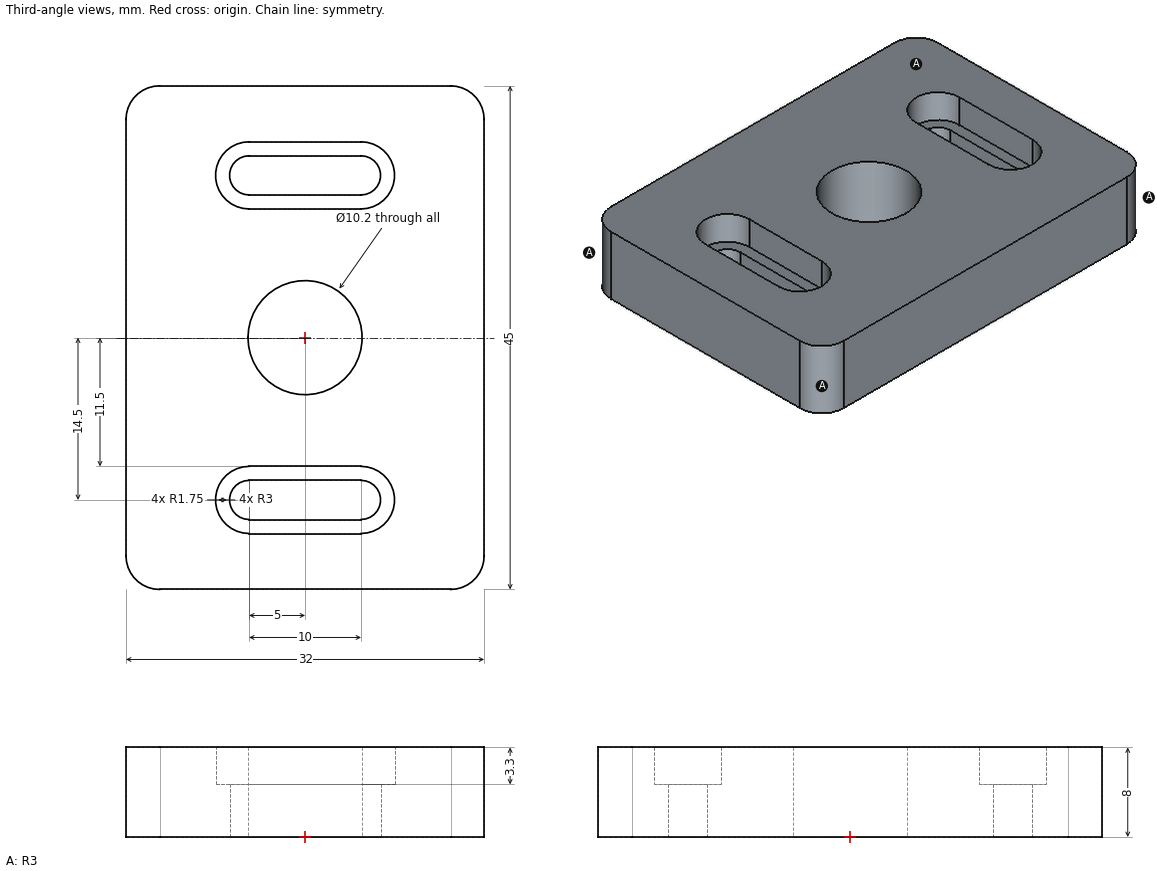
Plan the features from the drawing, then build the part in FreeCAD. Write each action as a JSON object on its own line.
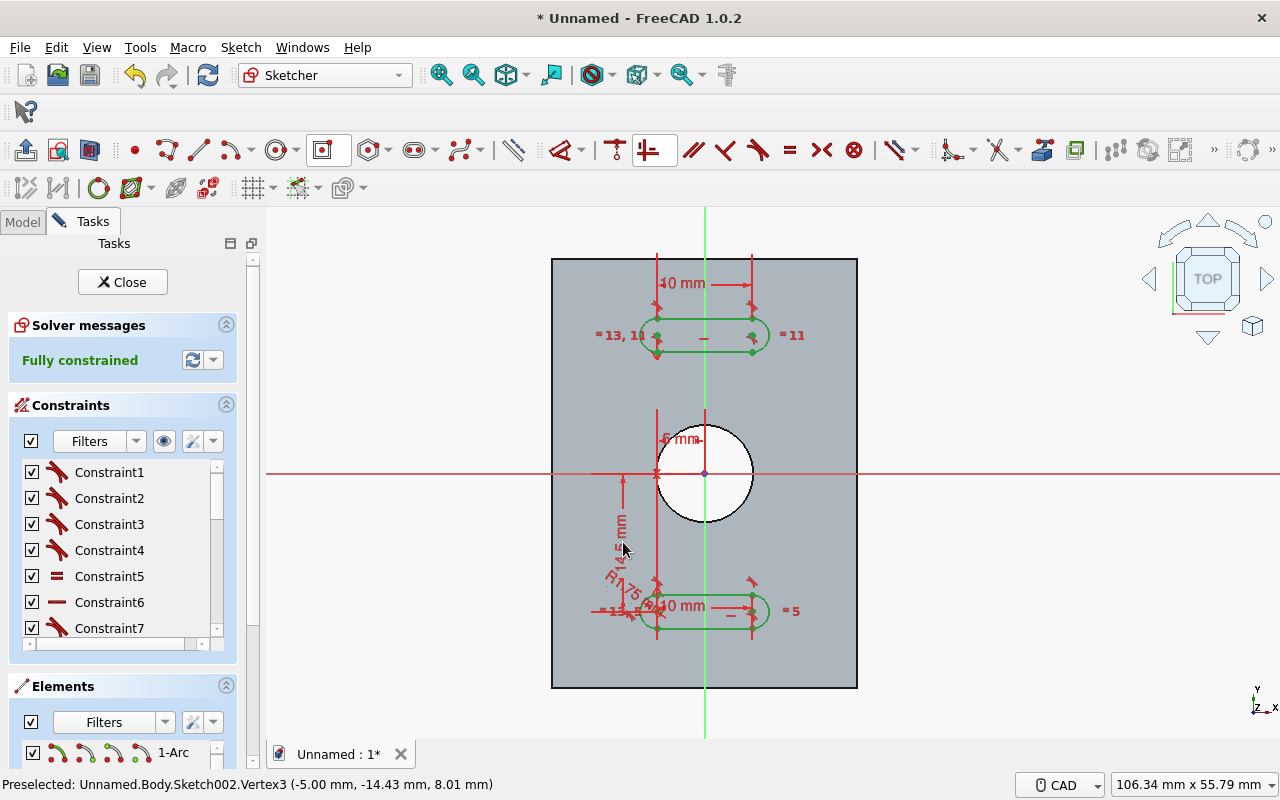
{"action": "left_click", "coordinate": [123, 282]}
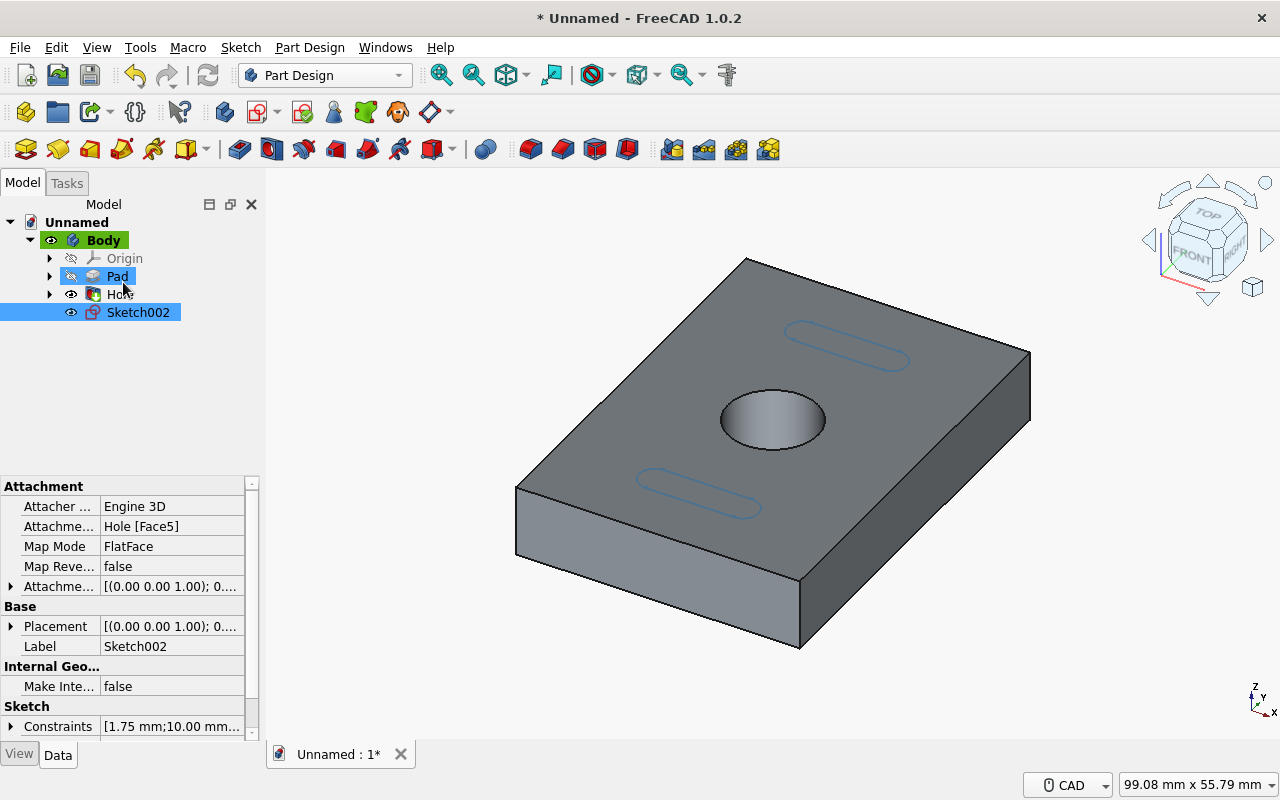
{"action": "left_click", "coordinate": [240, 150]}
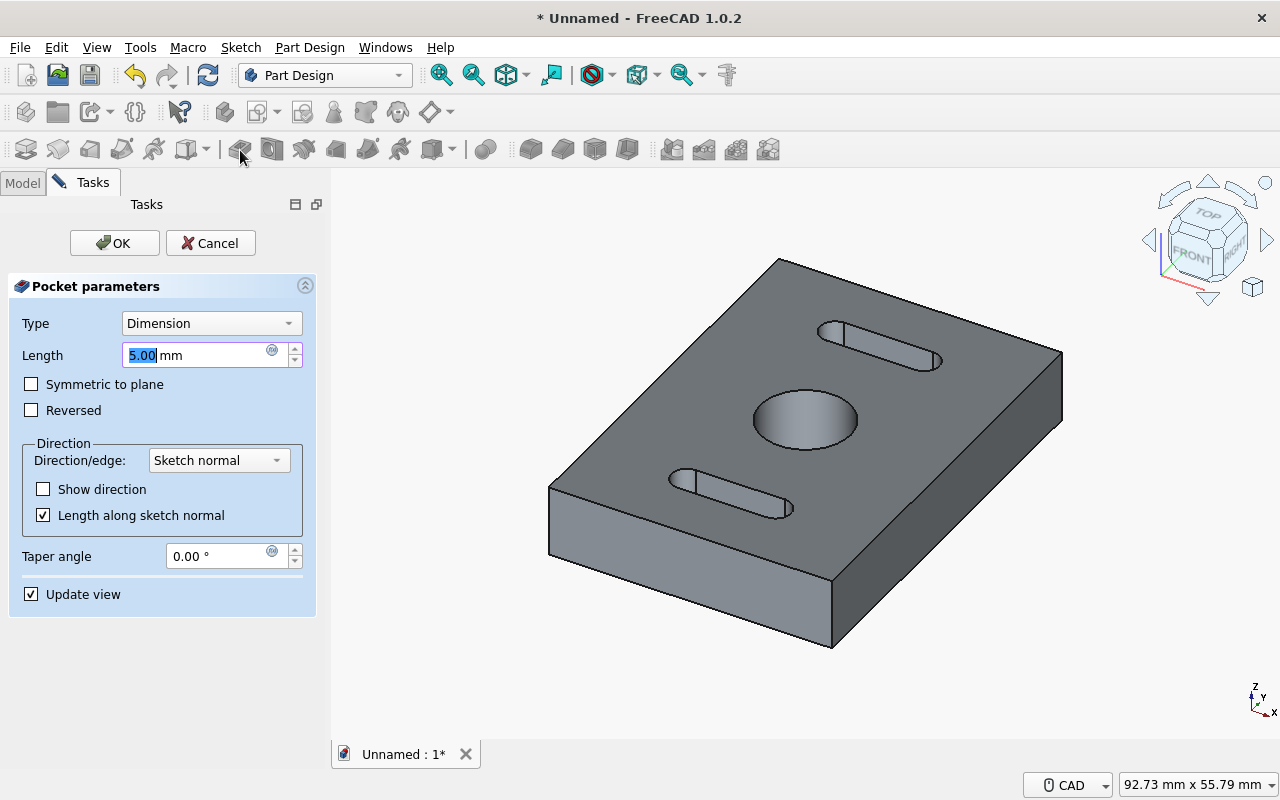
{"action": "left_click", "coordinate": [212, 324]}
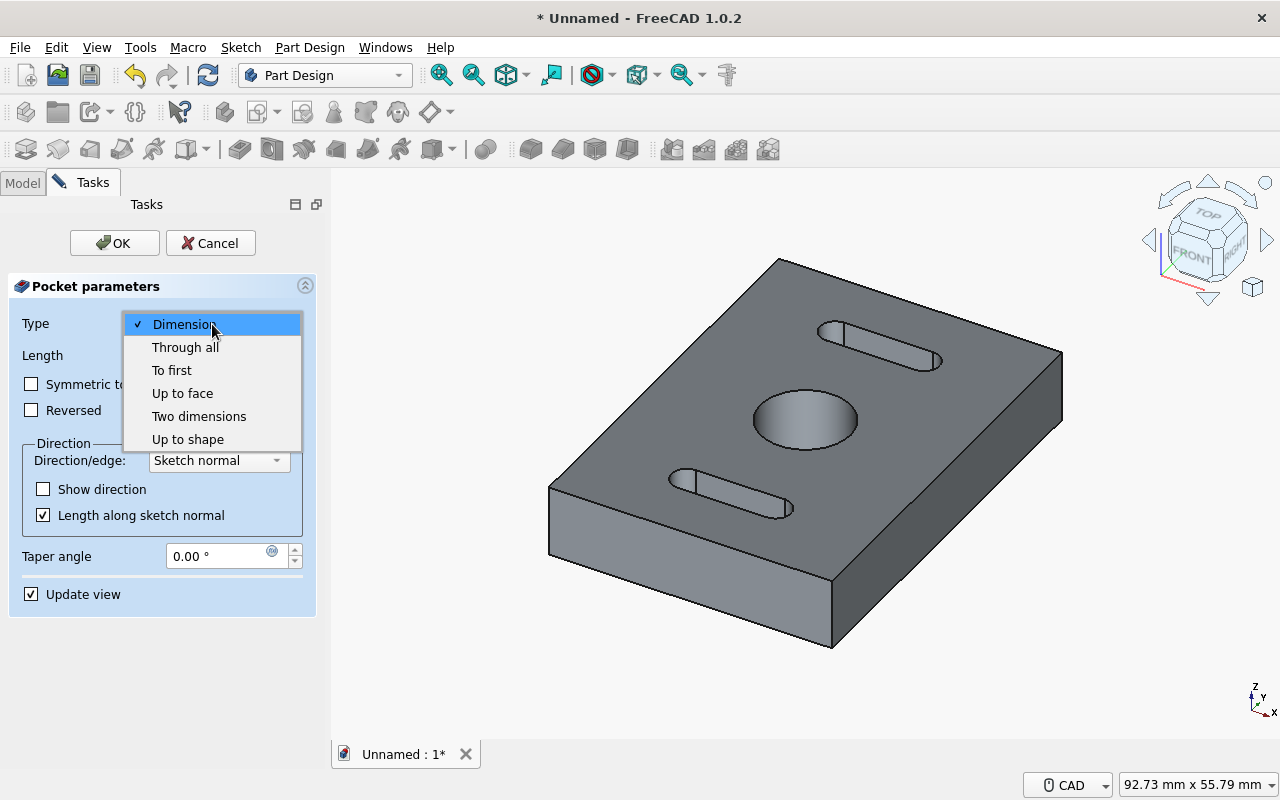
{"action": "left_click", "coordinate": [212, 348]}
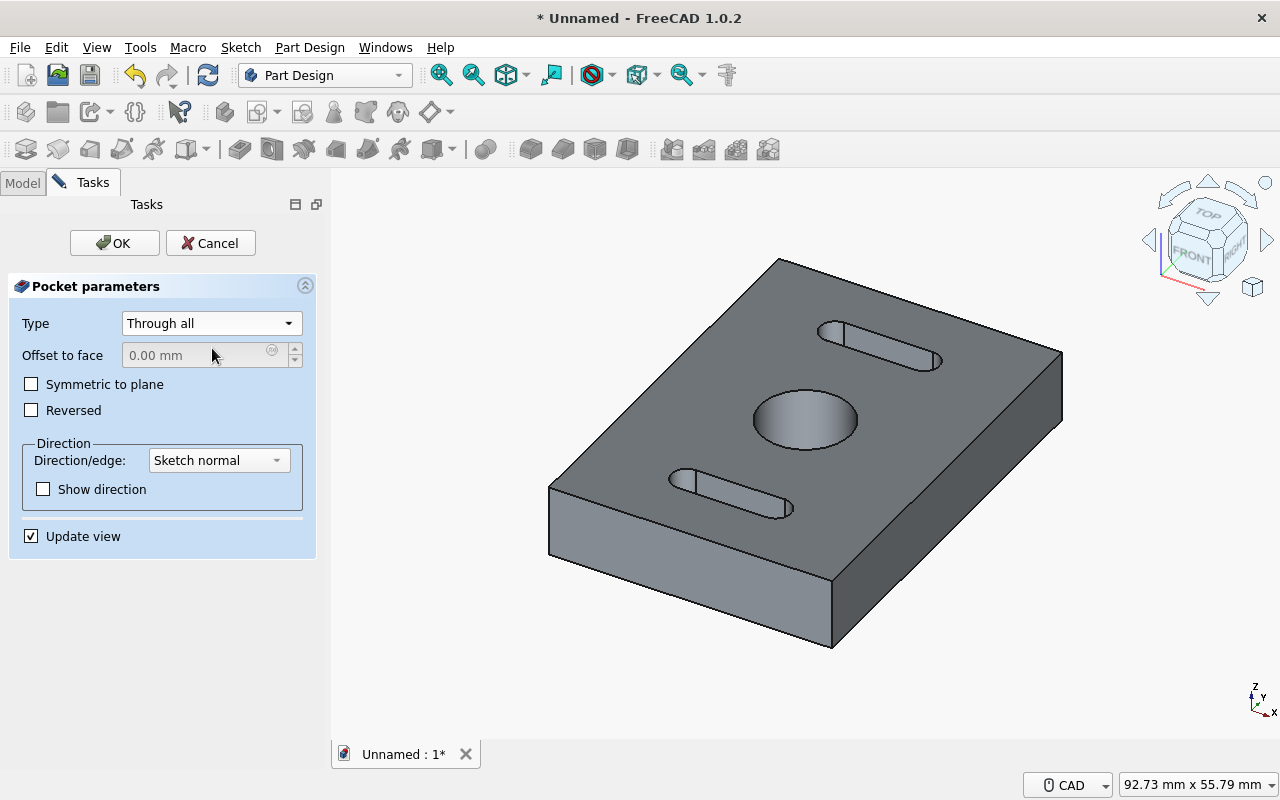
{"action": "left_click", "coordinate": [115, 243]}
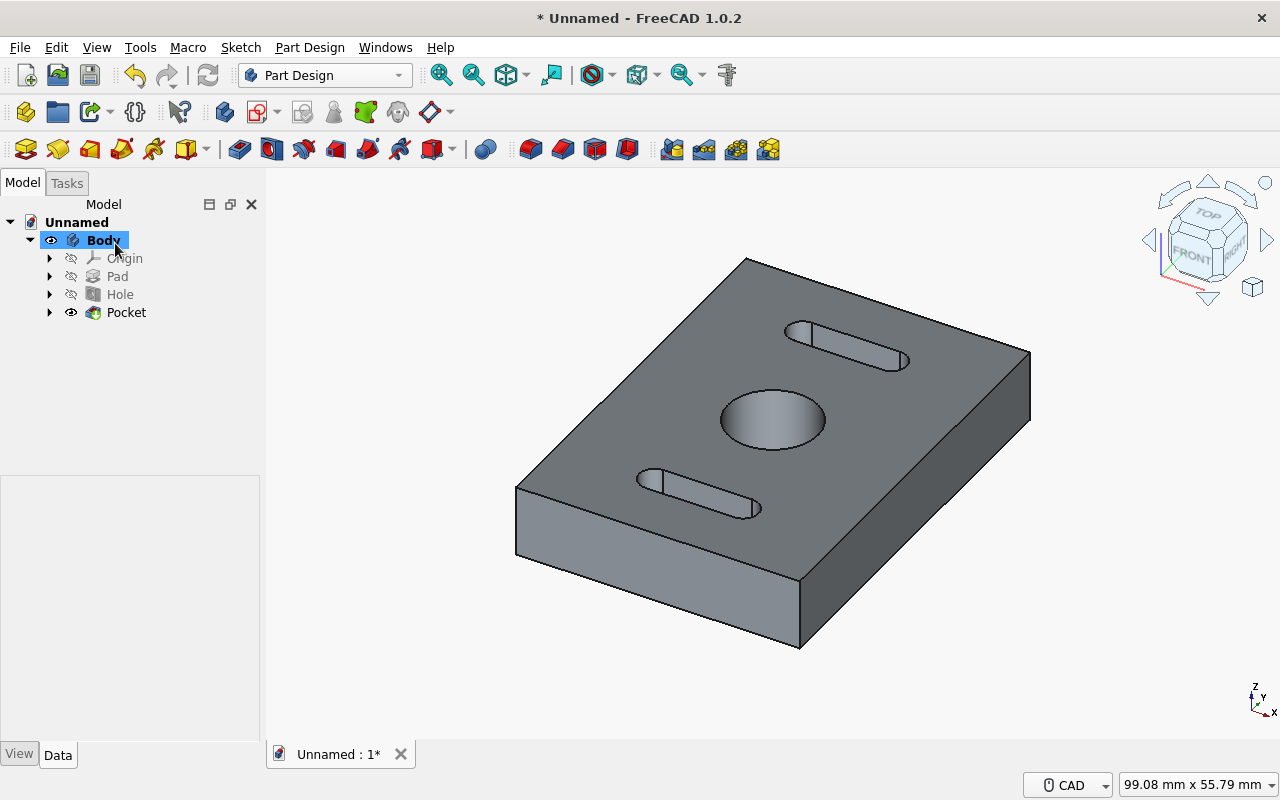
{"action": "left_click", "coordinate": [659, 425]}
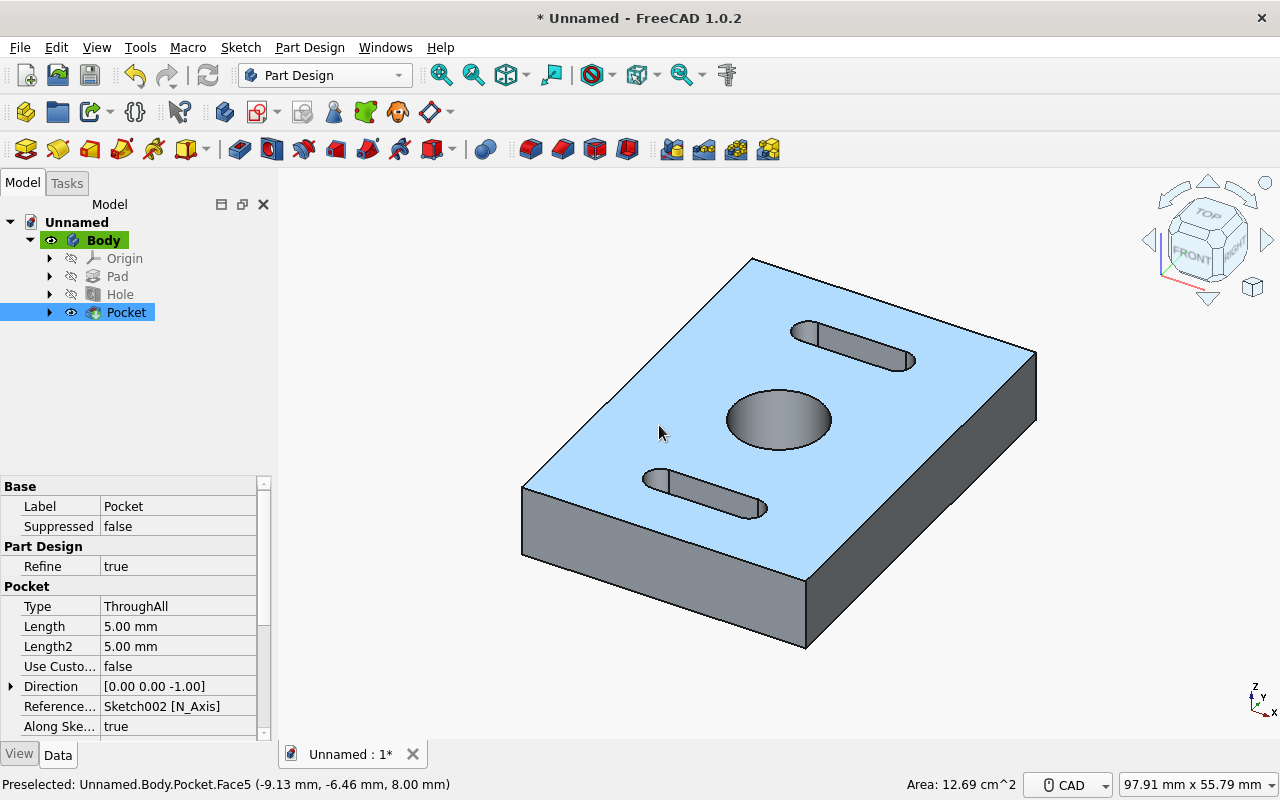
{"action": "left_click", "coordinate": [258, 112]}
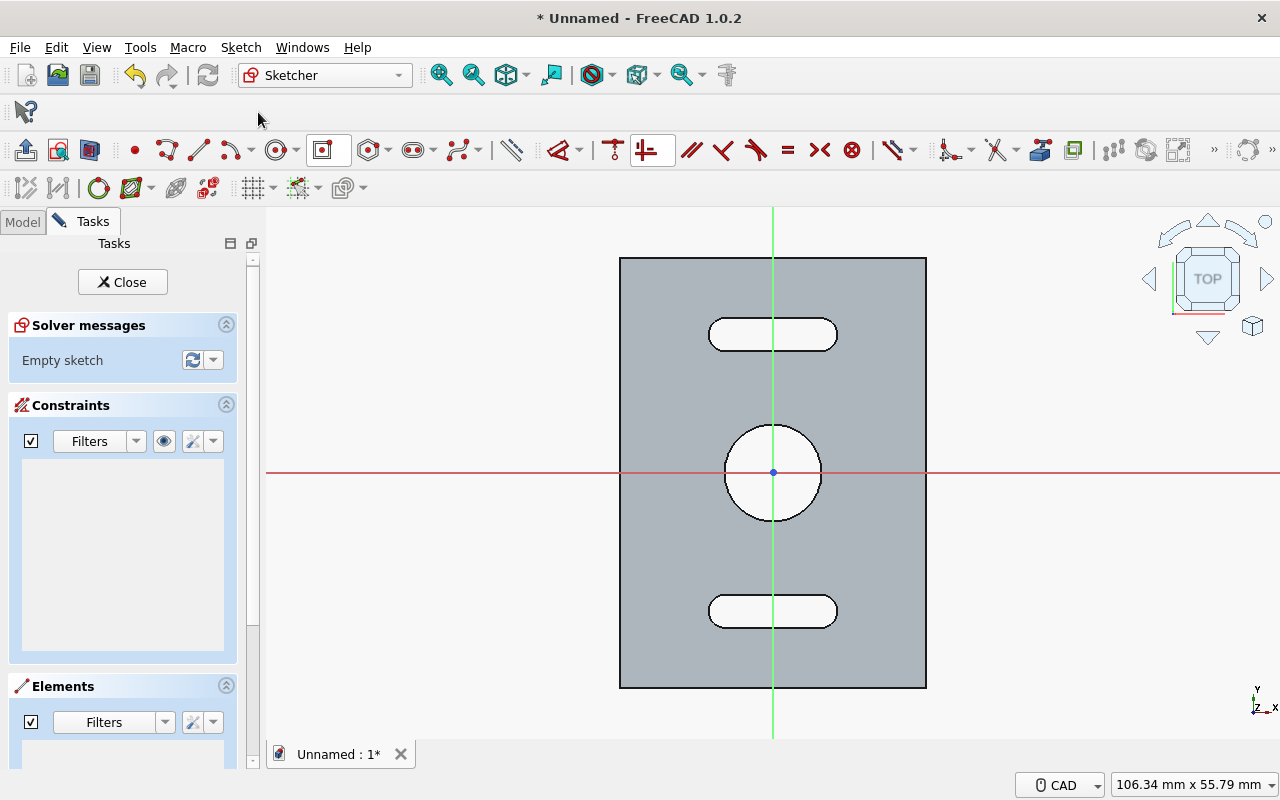
{"action": "left_click", "coordinate": [414, 150]}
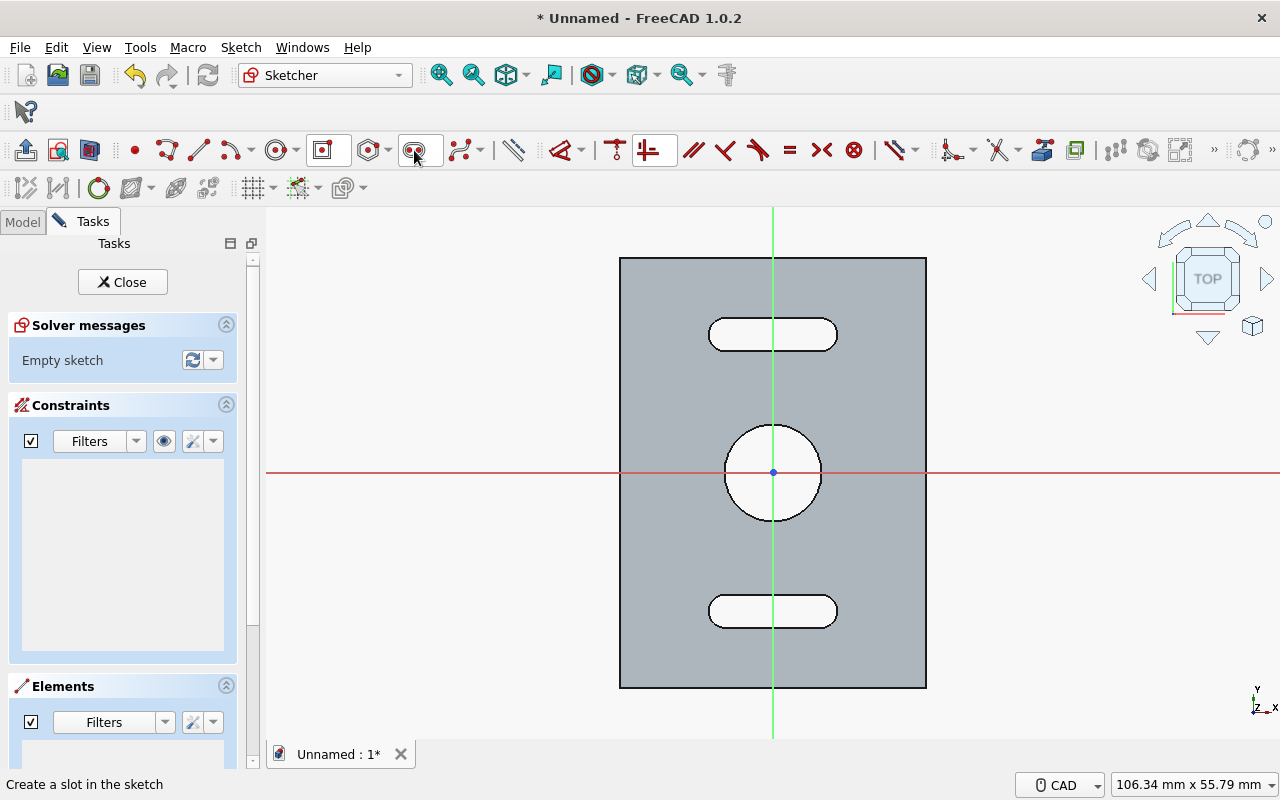
{"action": "left_click", "coordinate": [725, 611]}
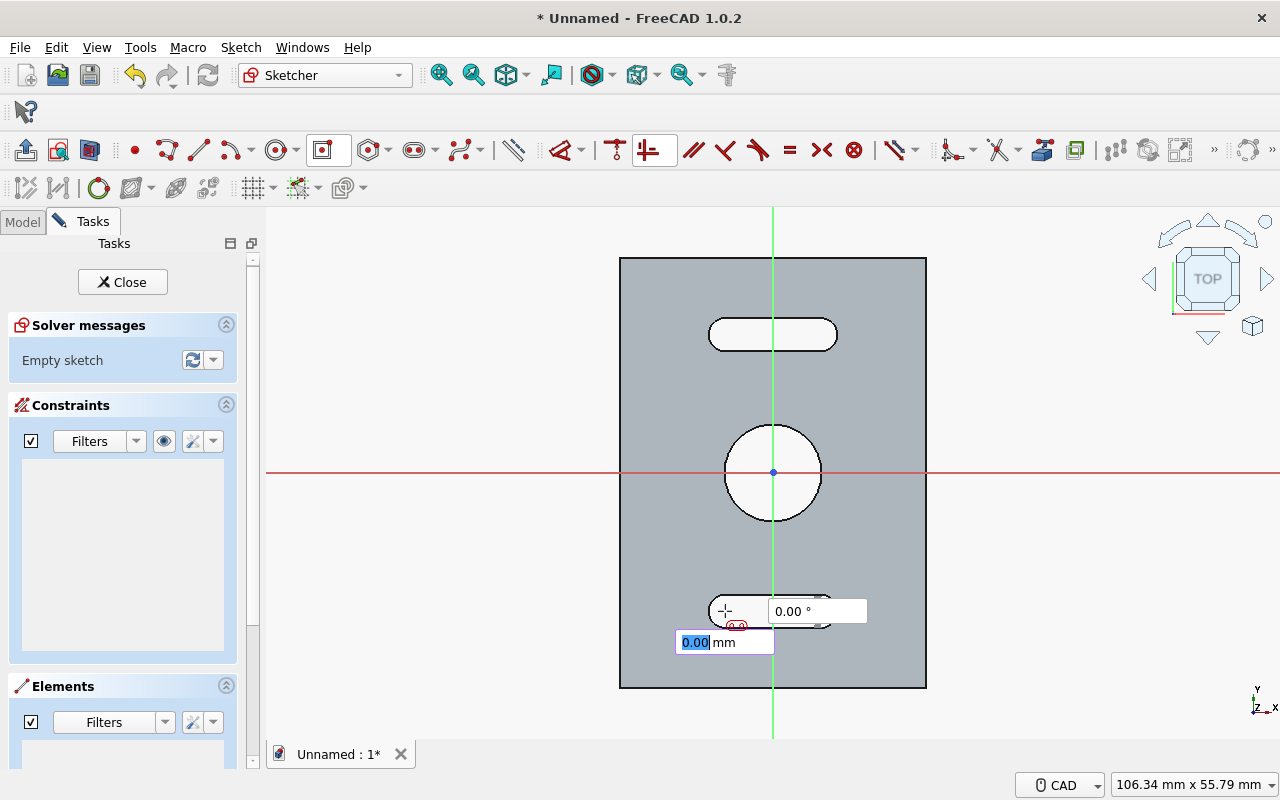
{"action": "left_click", "coordinate": [821, 611]}